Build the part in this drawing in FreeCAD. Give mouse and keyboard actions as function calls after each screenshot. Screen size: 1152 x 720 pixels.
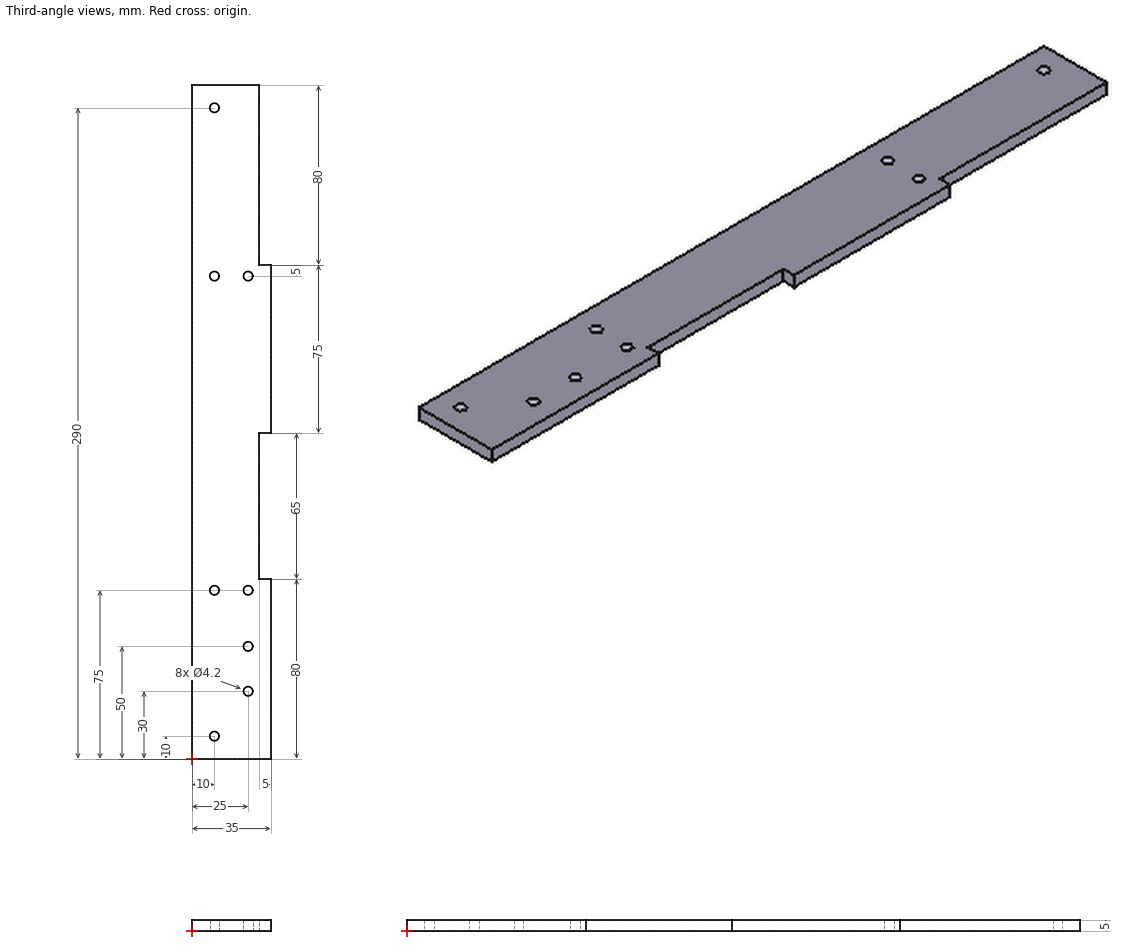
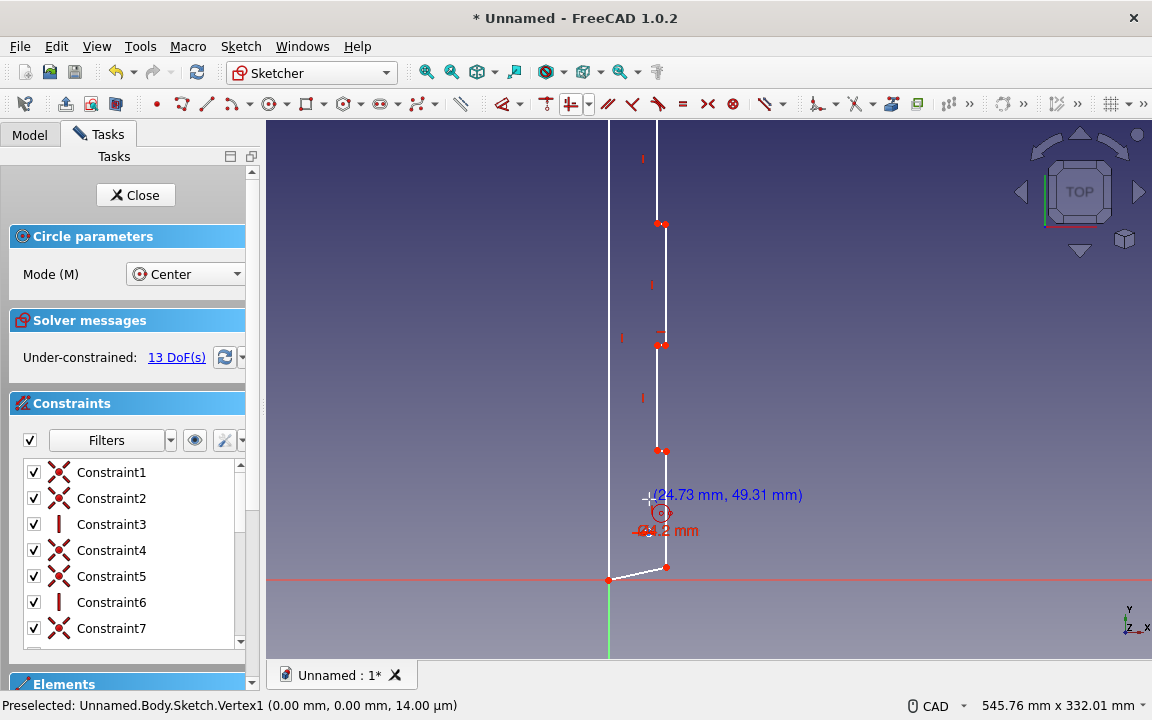
click(649, 499)
move(647, 497)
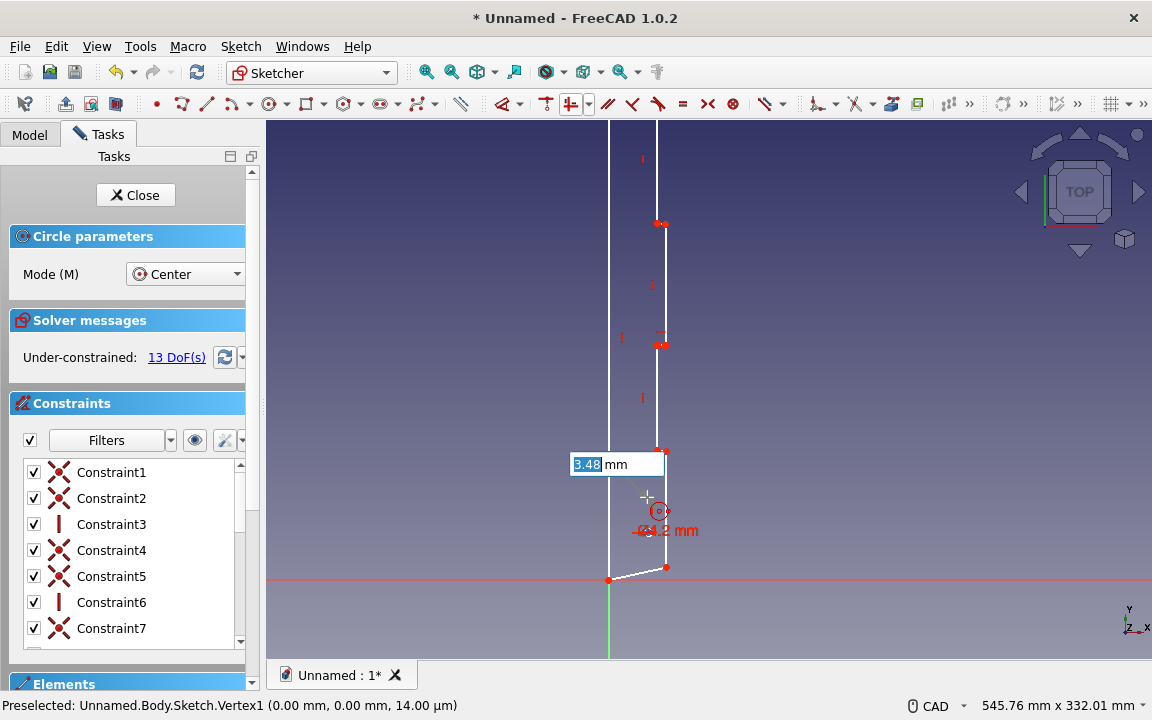
text(4.2)
key(Return)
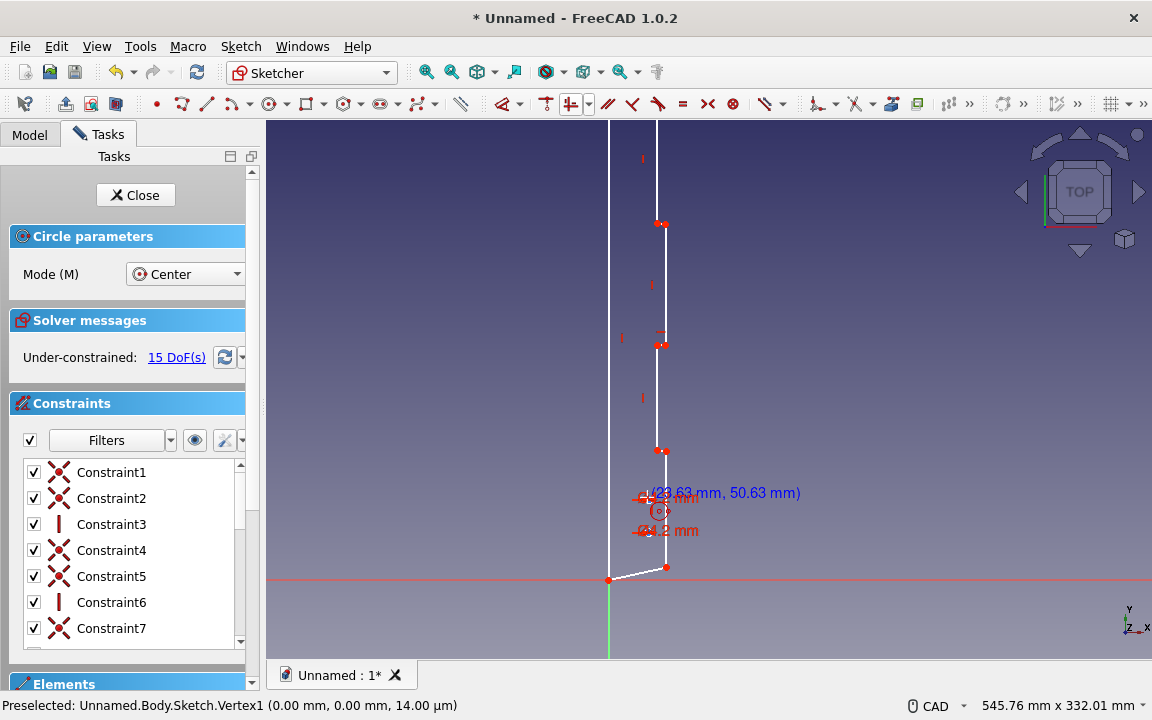
scroll(649, 458, up, 10)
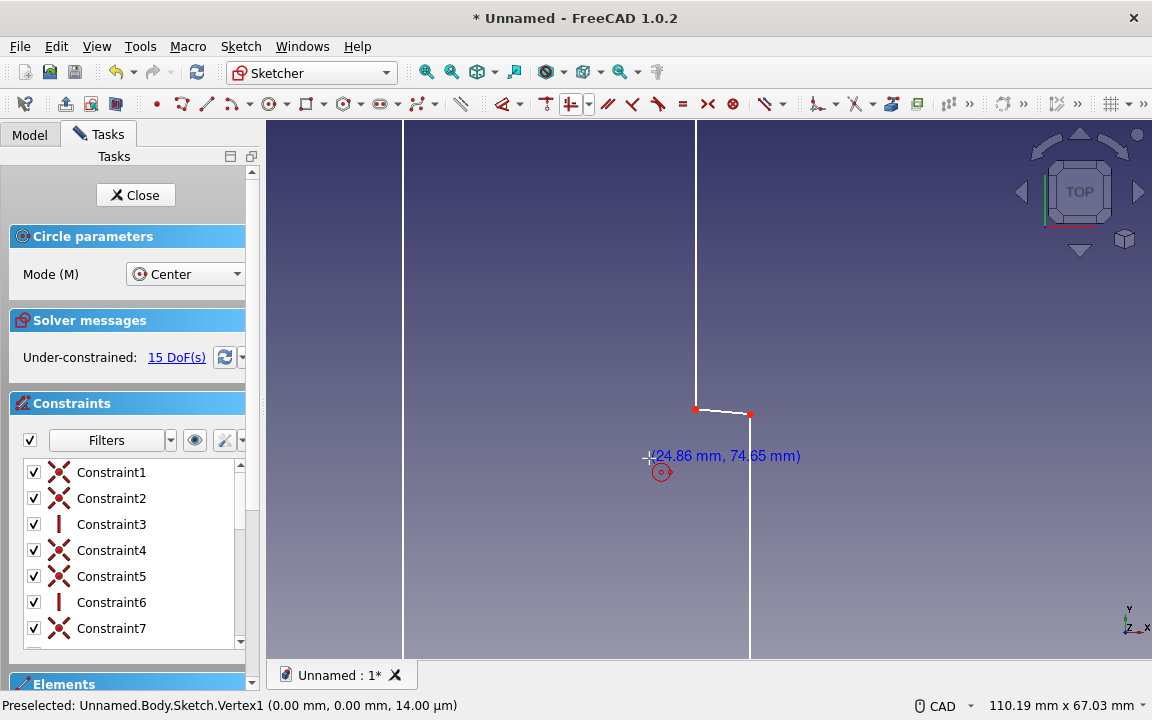
scroll(649, 473, down, 12)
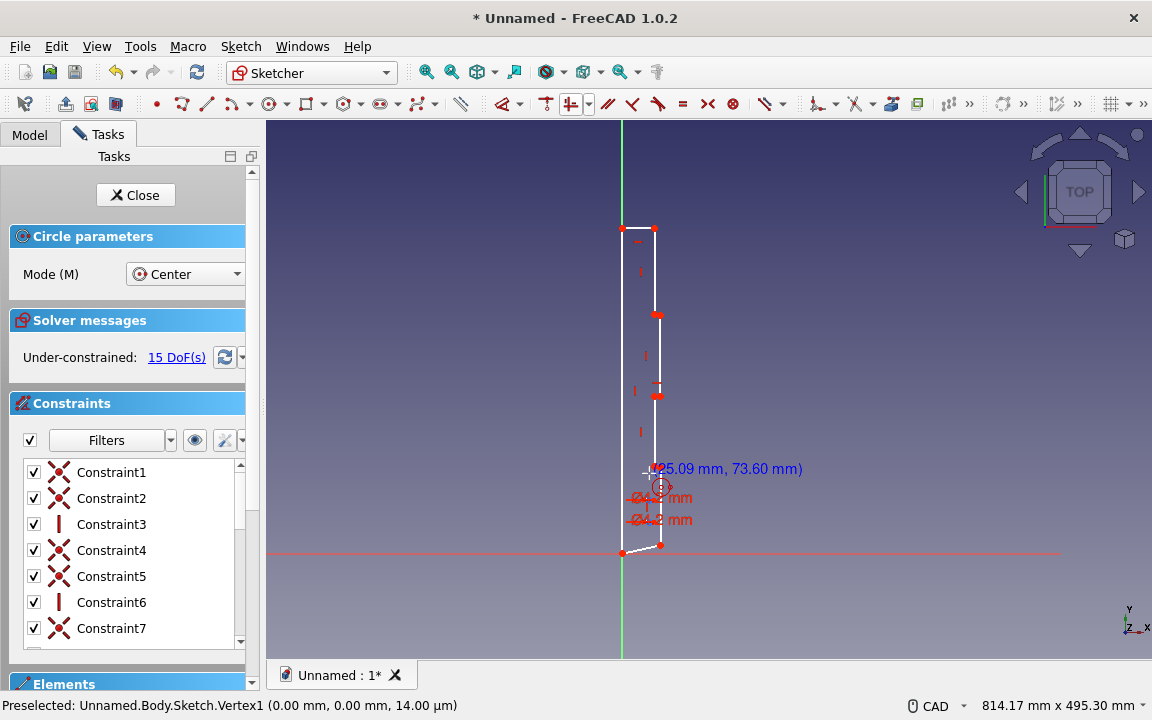
scroll(649, 472, up, 4)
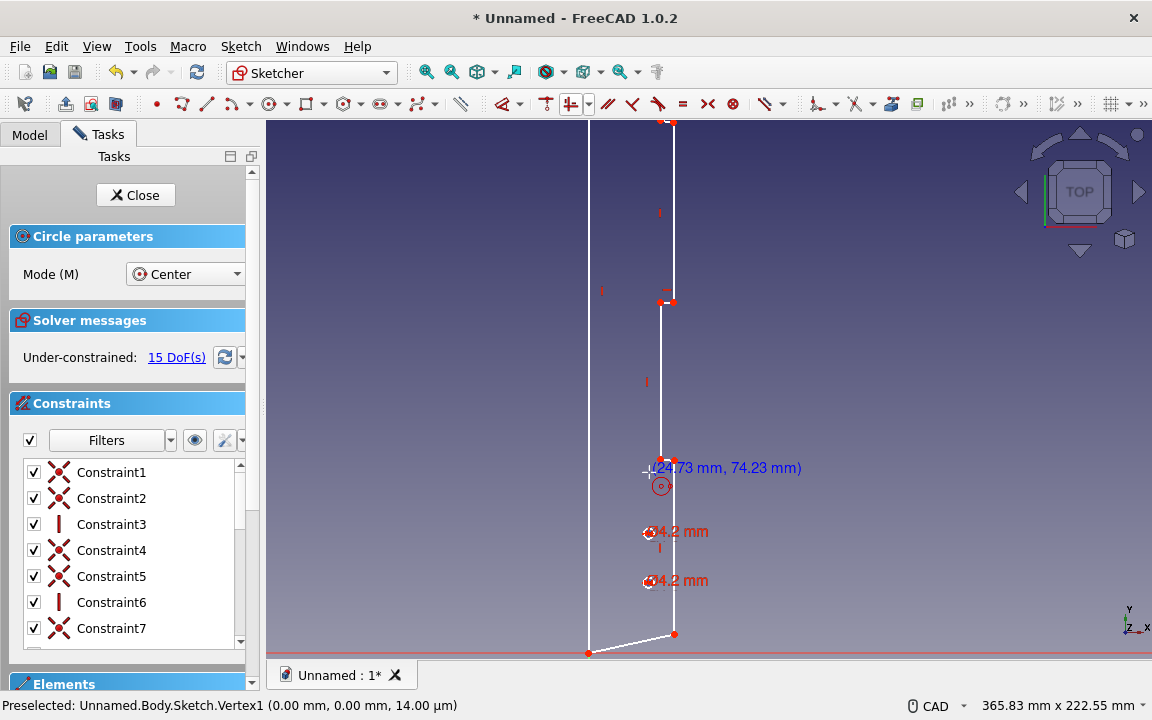
click(649, 472)
move(646, 468)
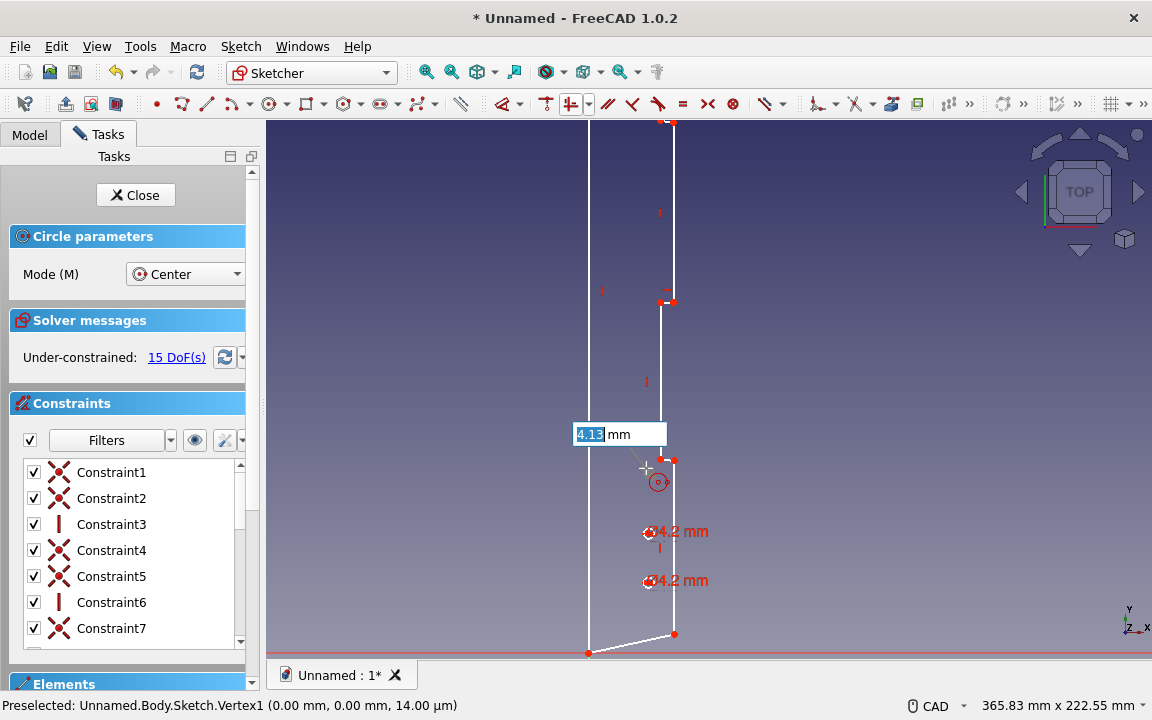
text(4.2)
key(Return)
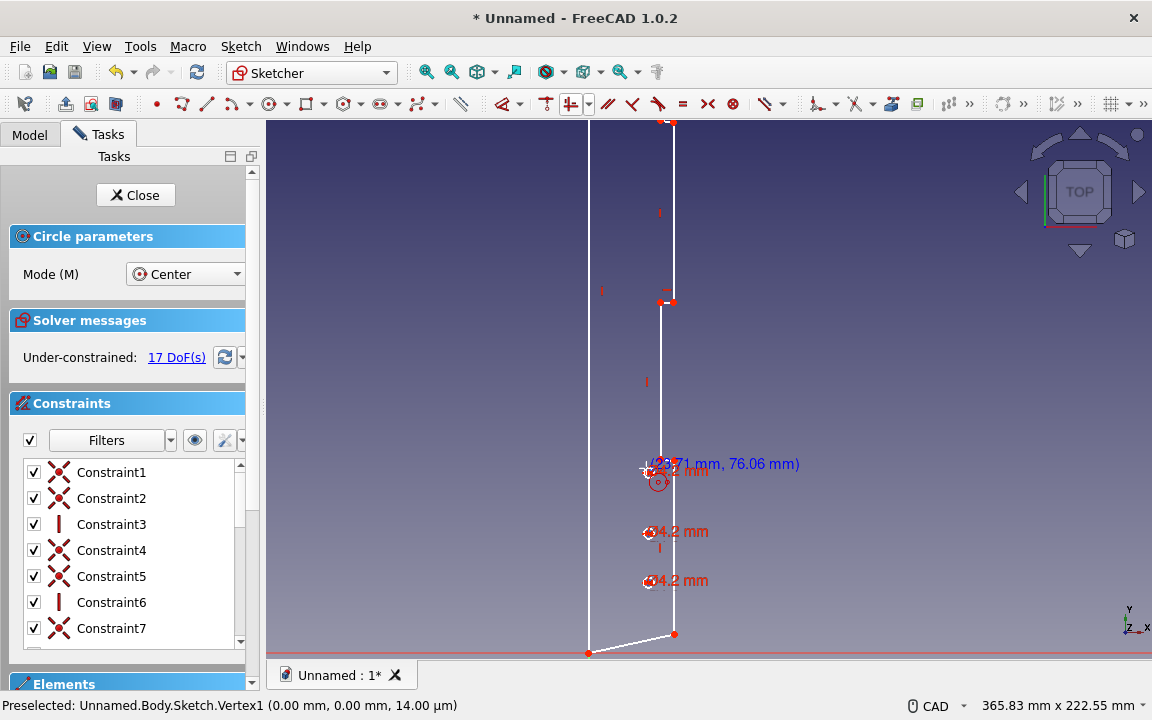
scroll(613, 629, up, 8)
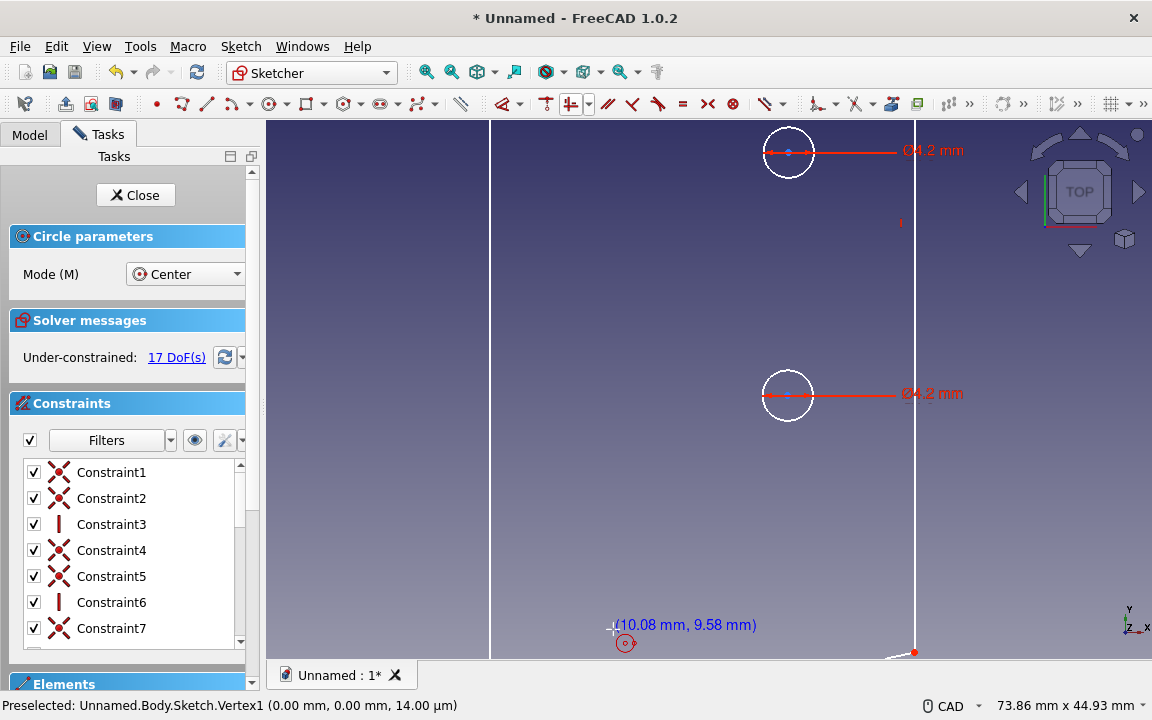
scroll(635, 534, down, 12)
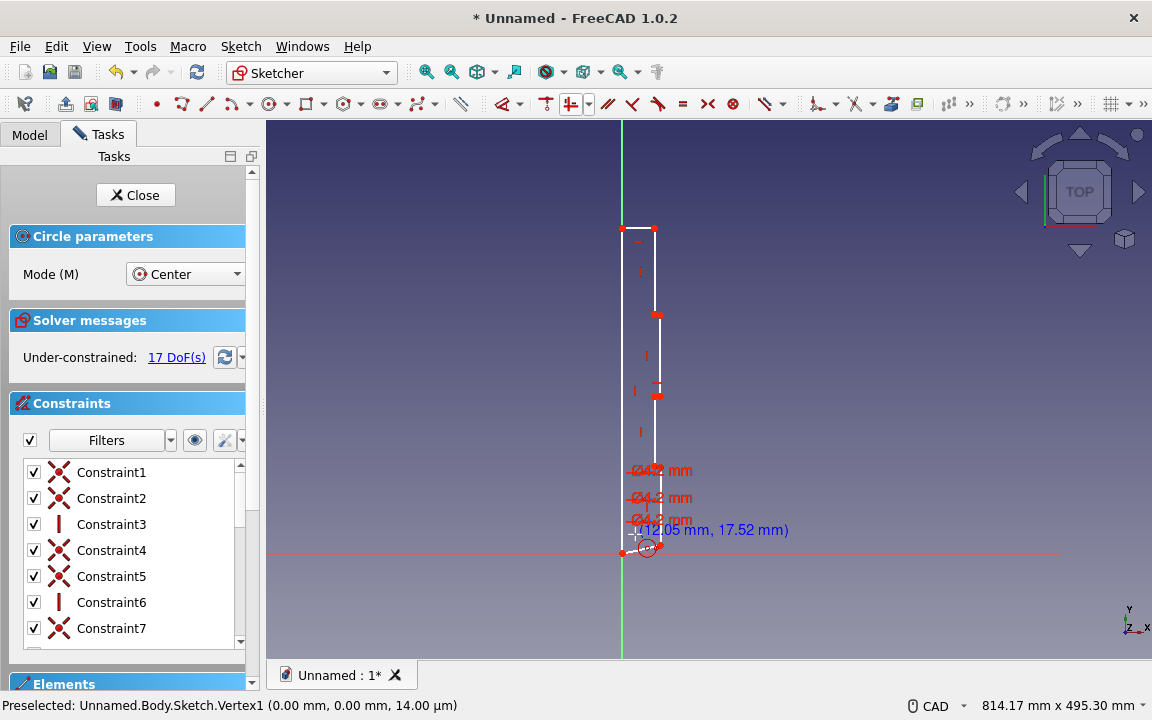
scroll(633, 543, up, 2)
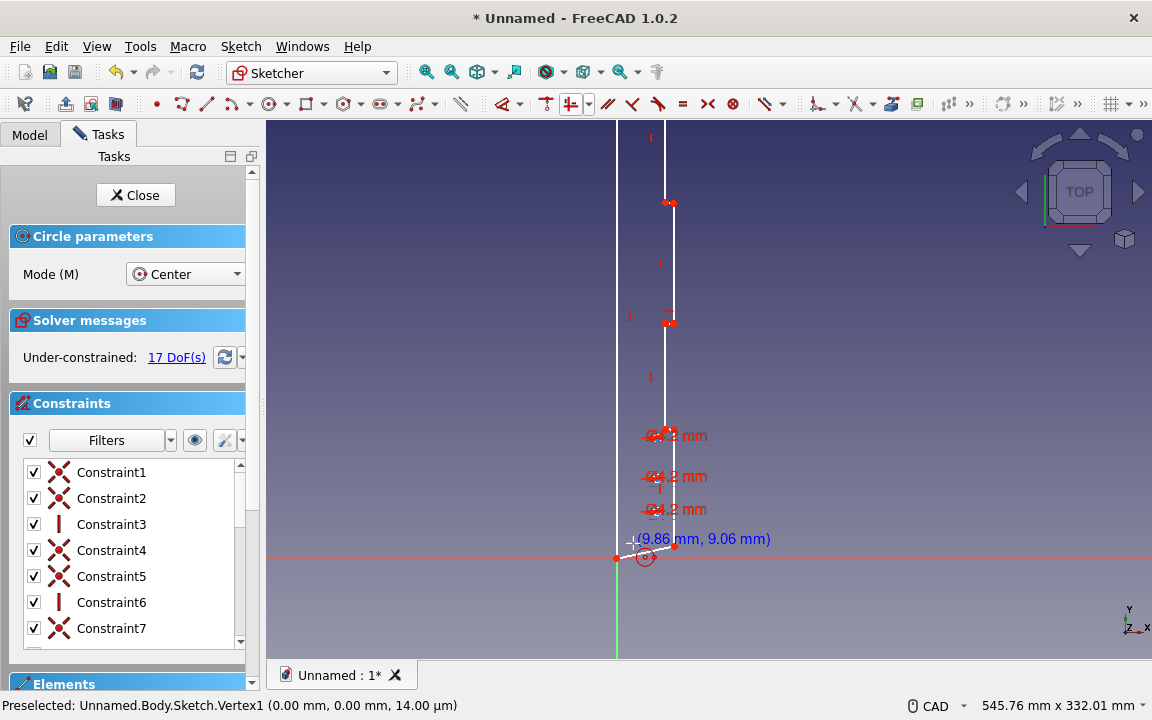
click(633, 543)
move(635, 540)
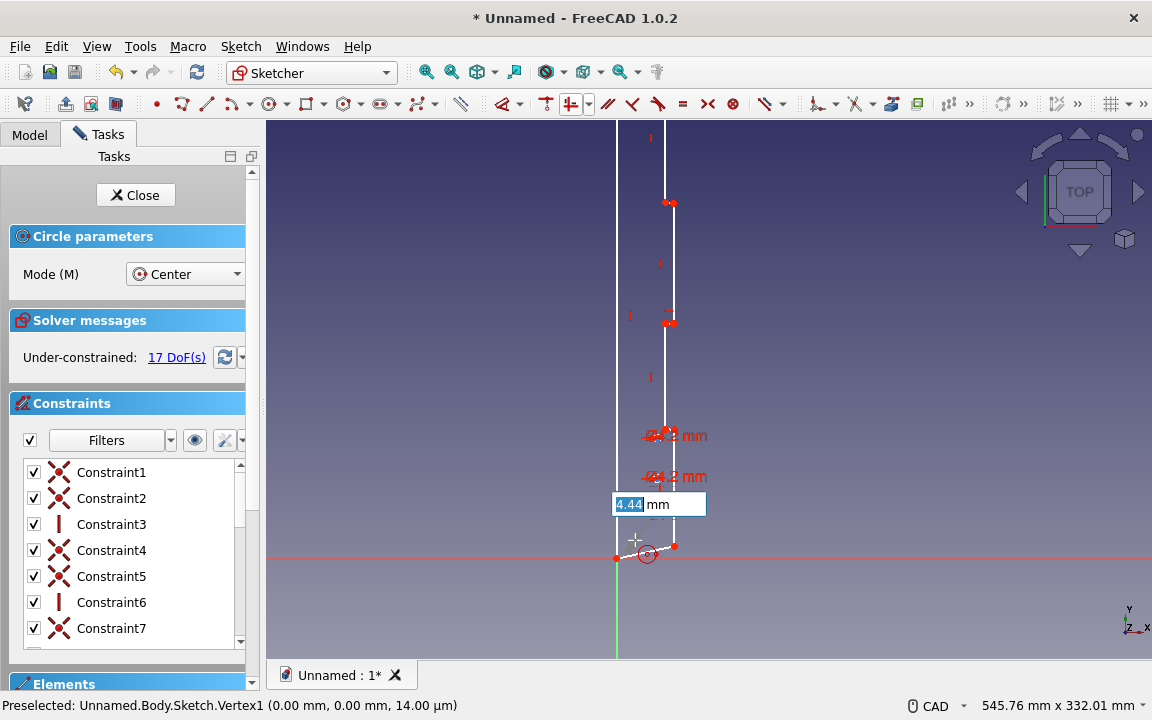
text(4.2)
key(Return)